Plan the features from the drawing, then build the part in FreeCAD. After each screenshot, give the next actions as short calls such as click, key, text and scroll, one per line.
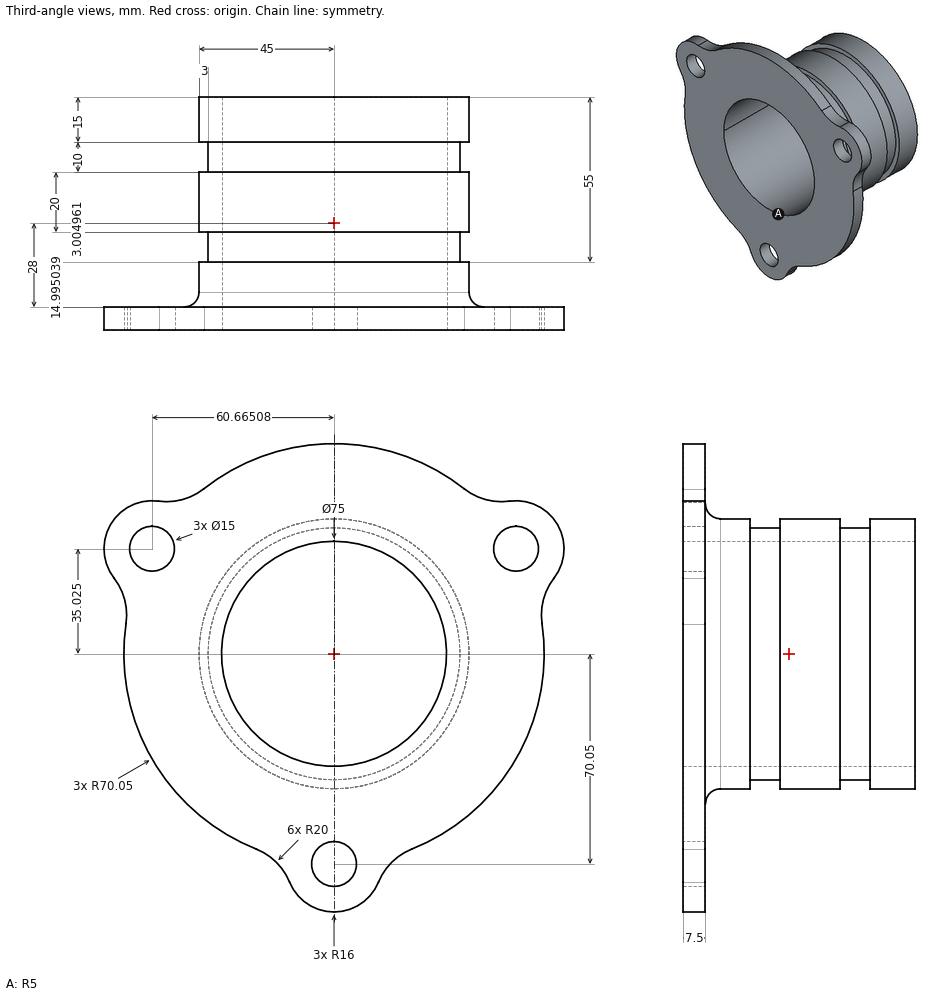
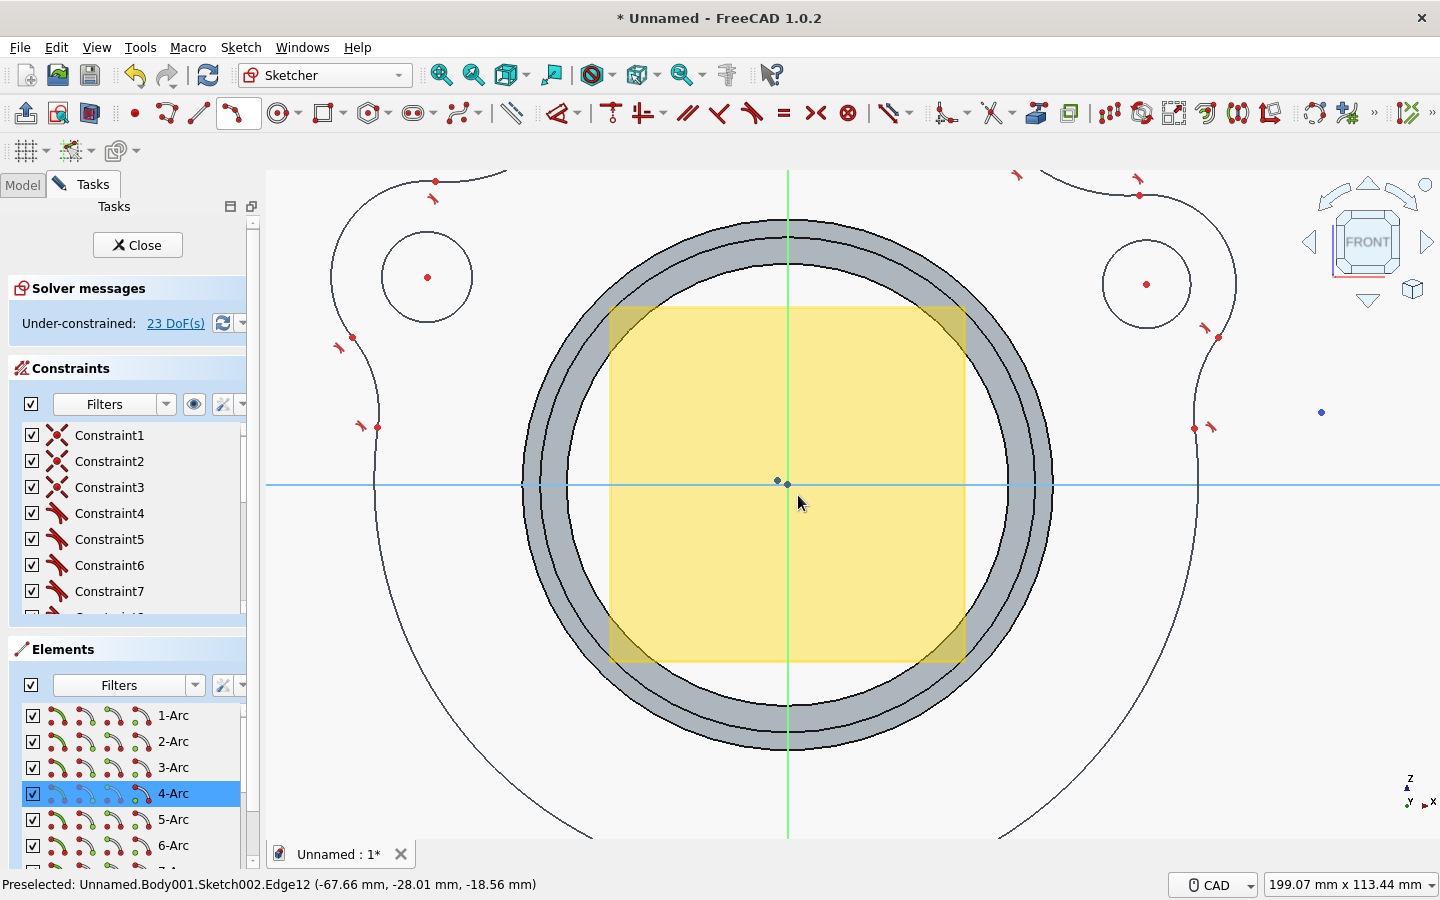
key(c)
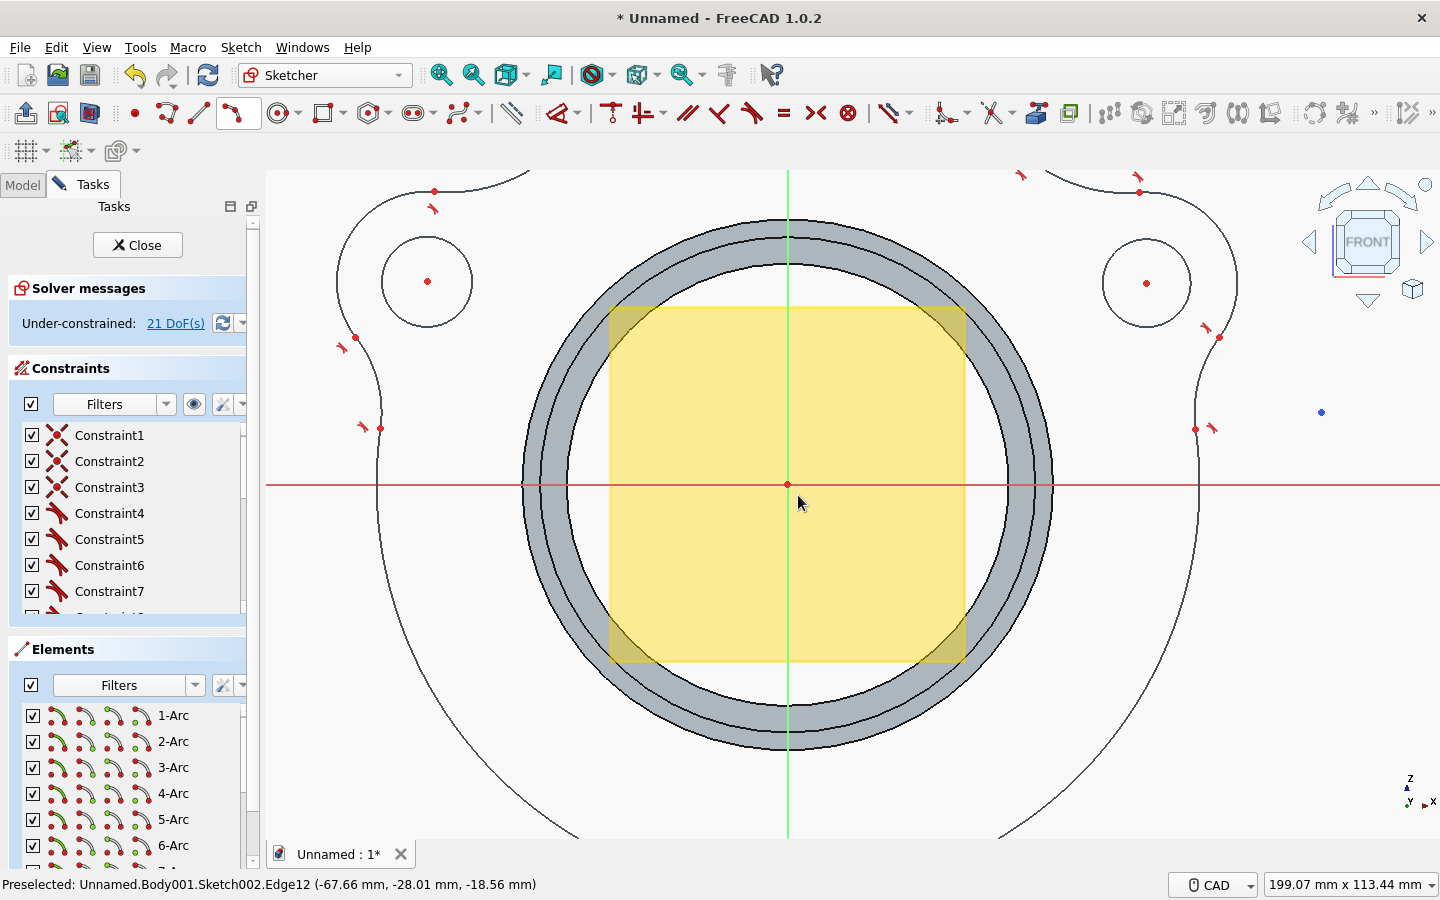
click(381, 400)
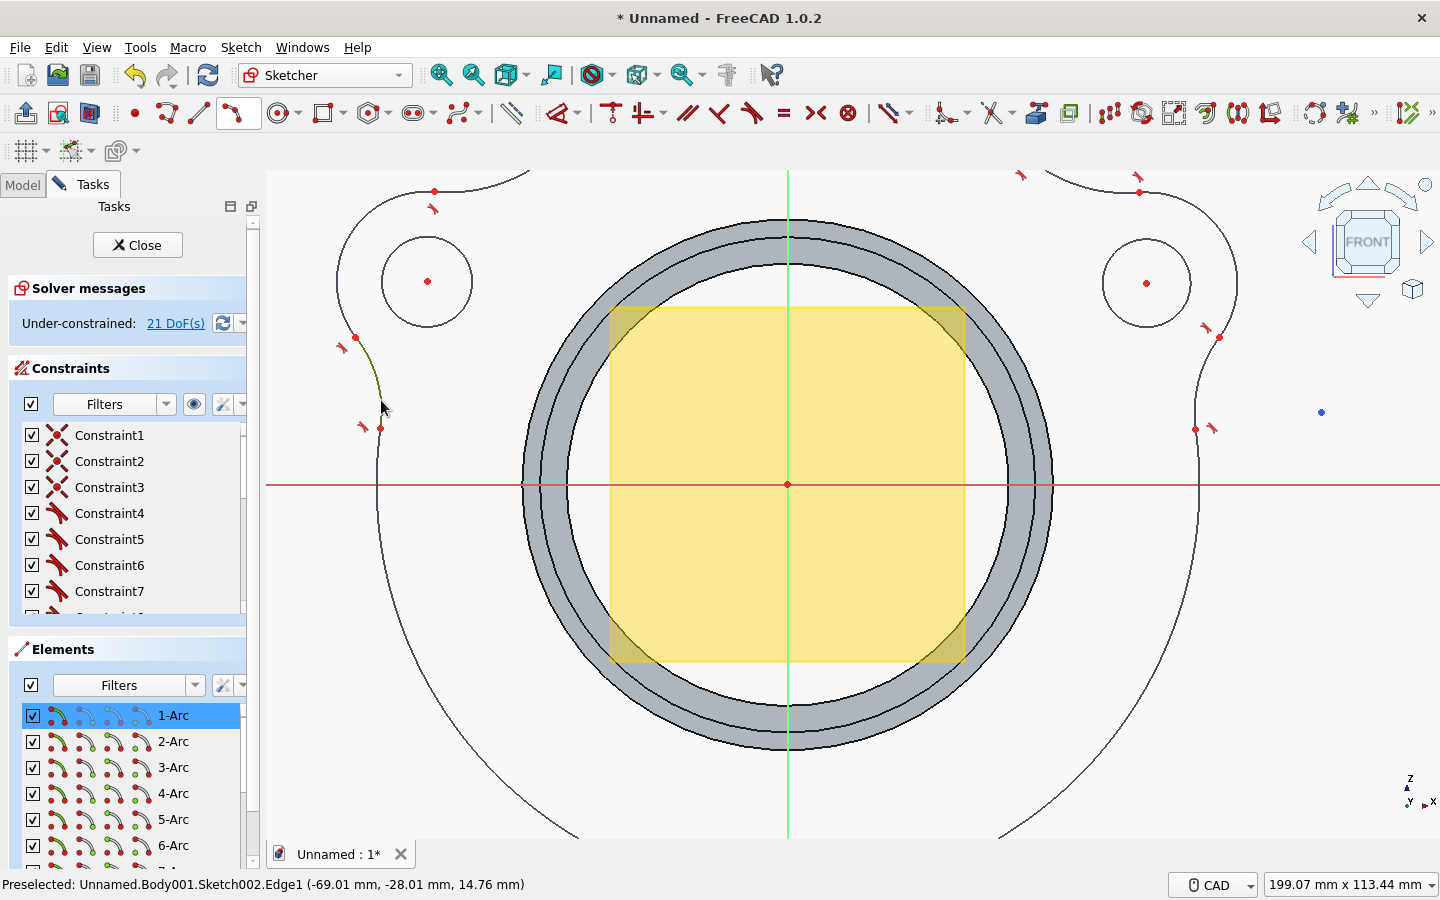
scroll(782, 482, down, 4)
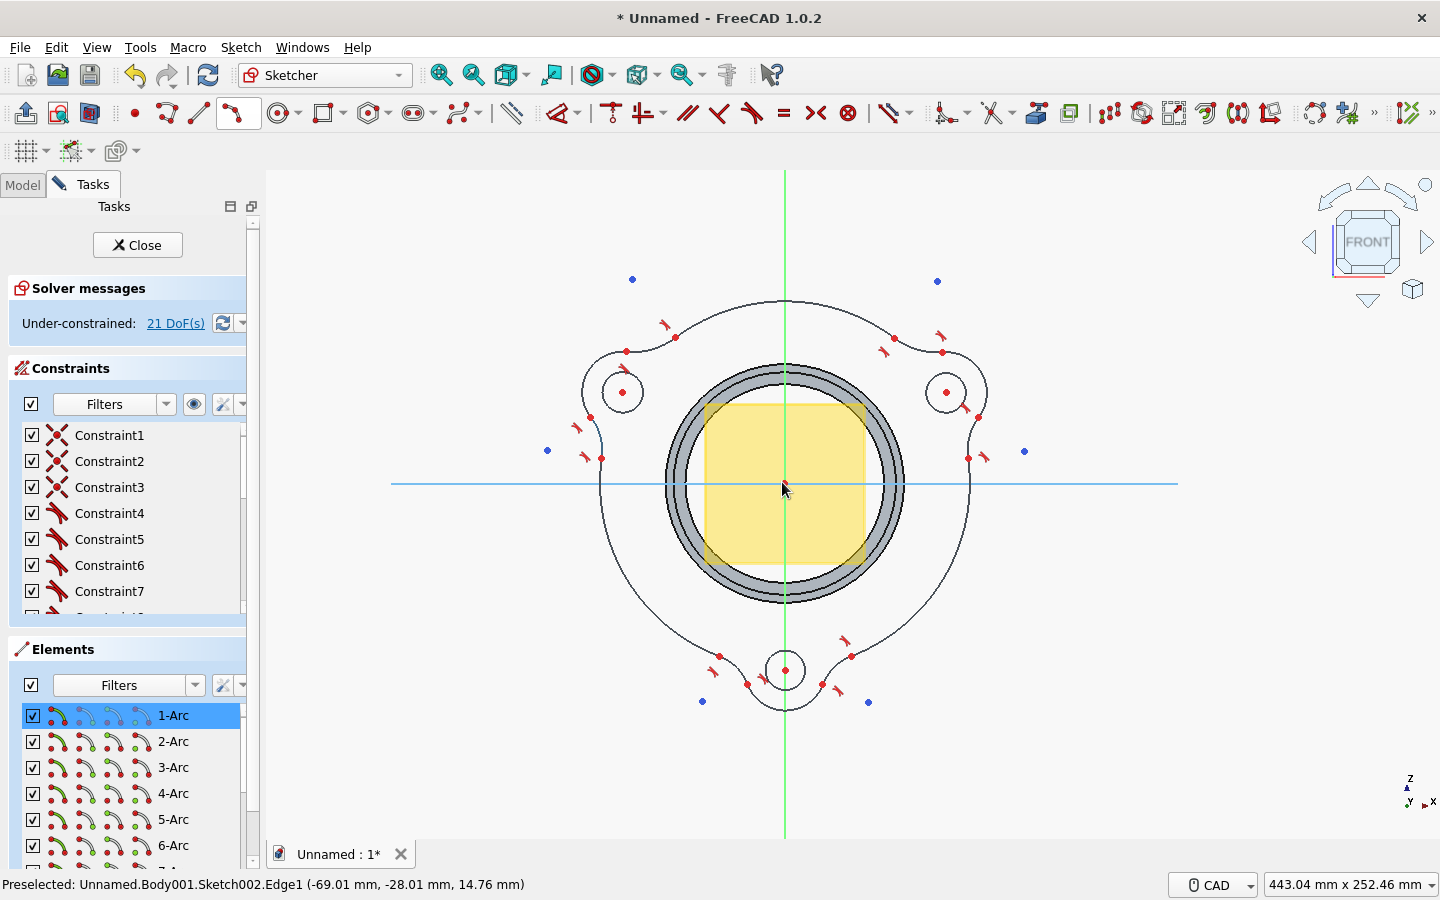
click(642, 352)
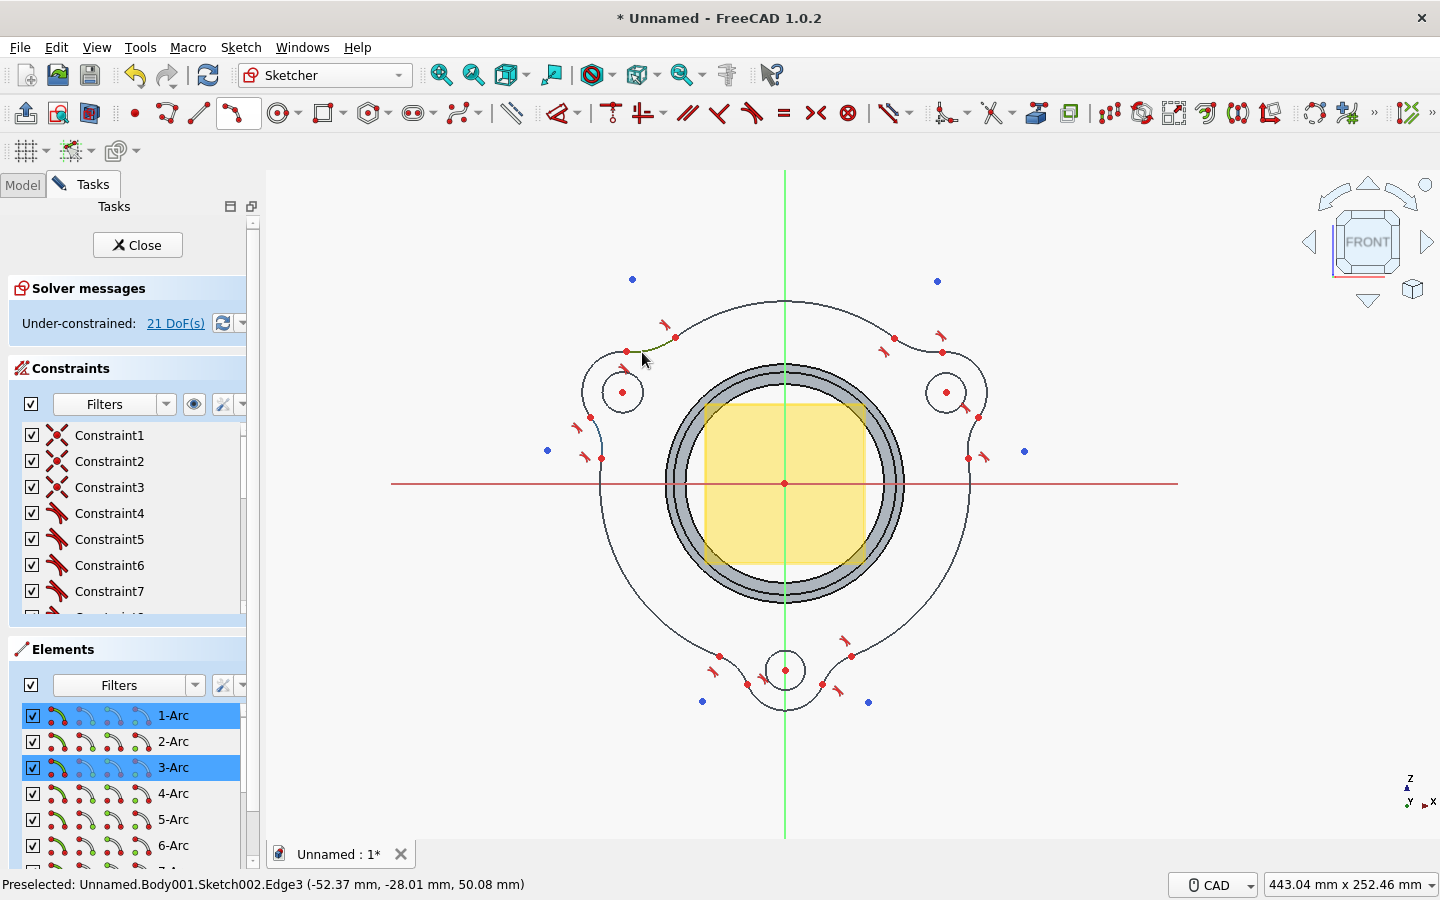
click(908, 346)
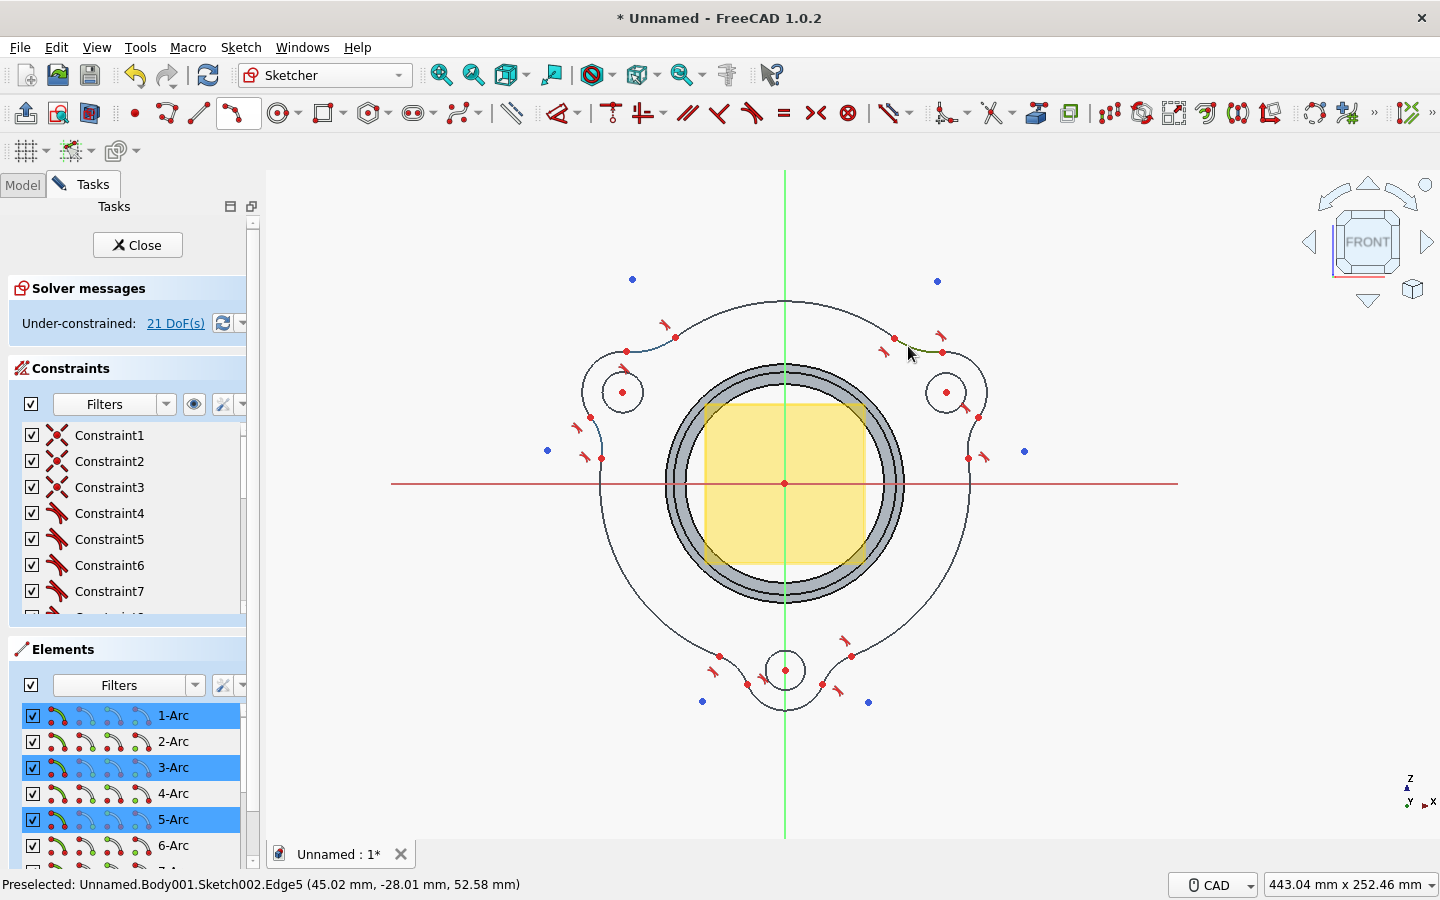
click(972, 429)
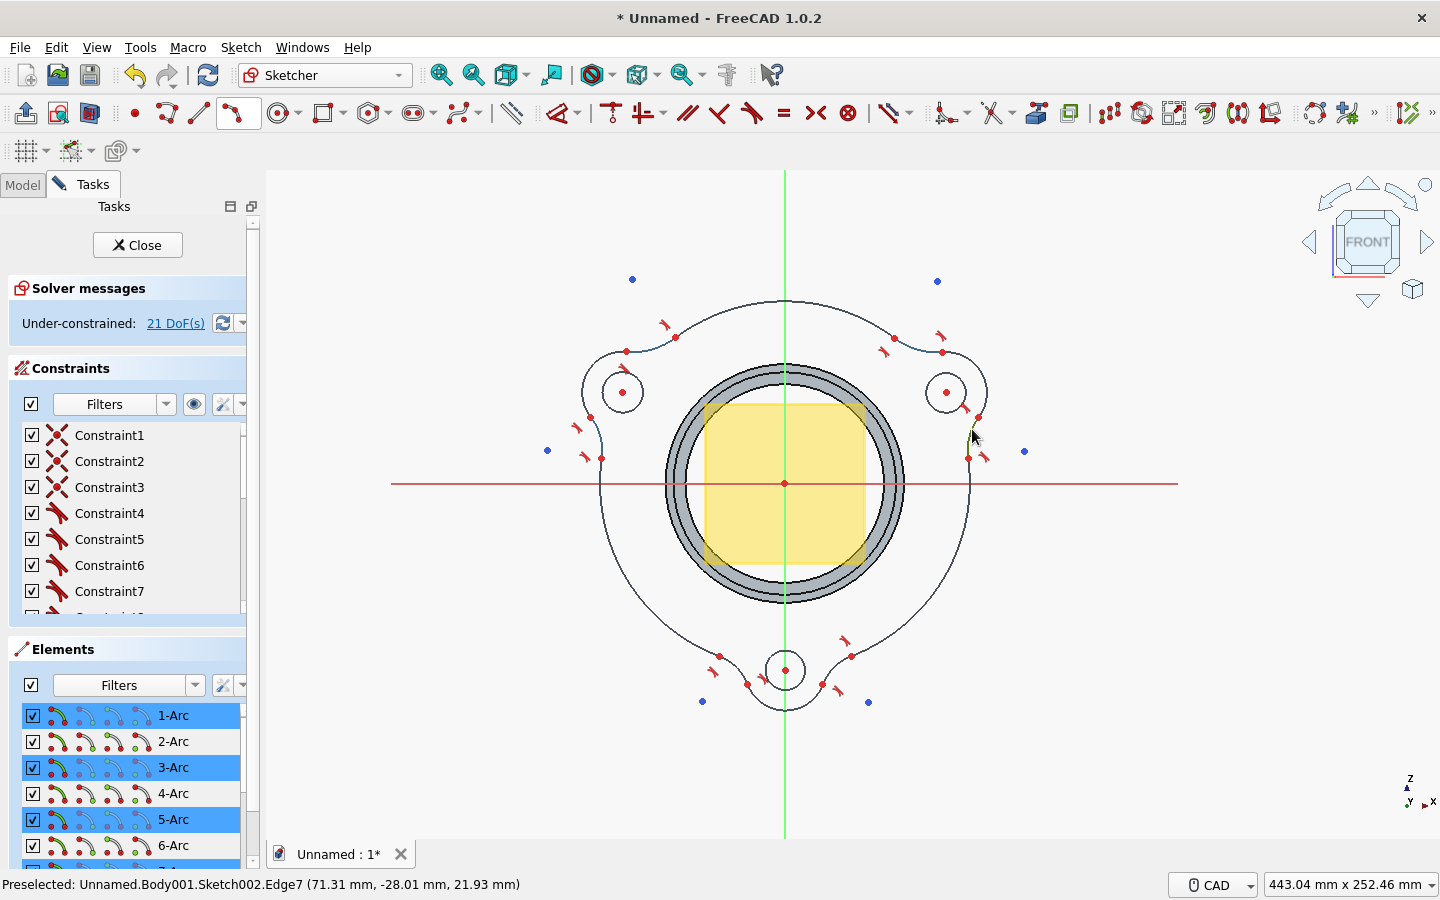
click(840, 662)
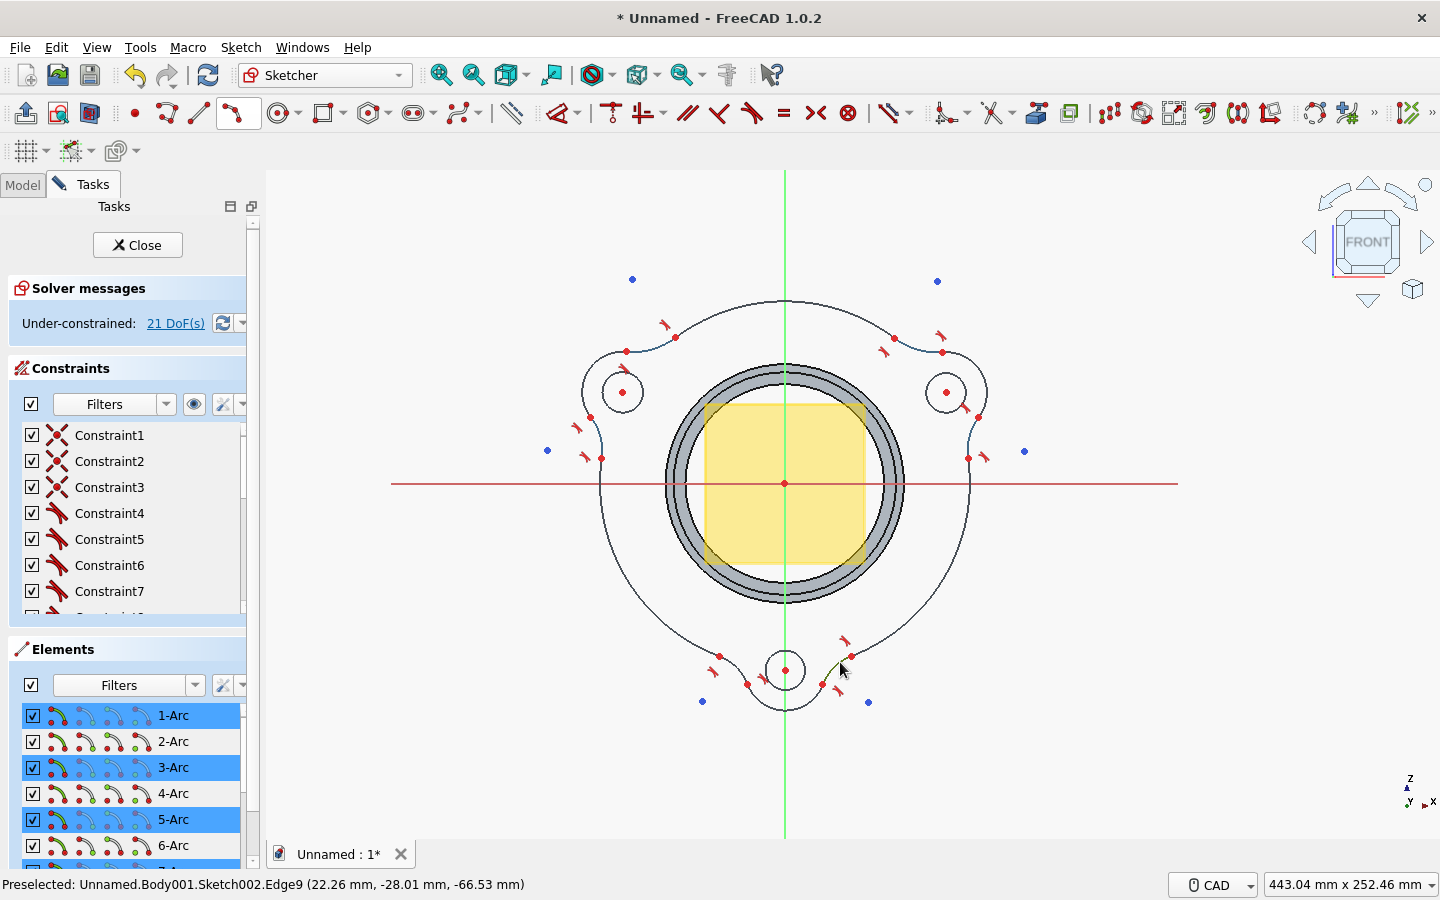
click(742, 674)